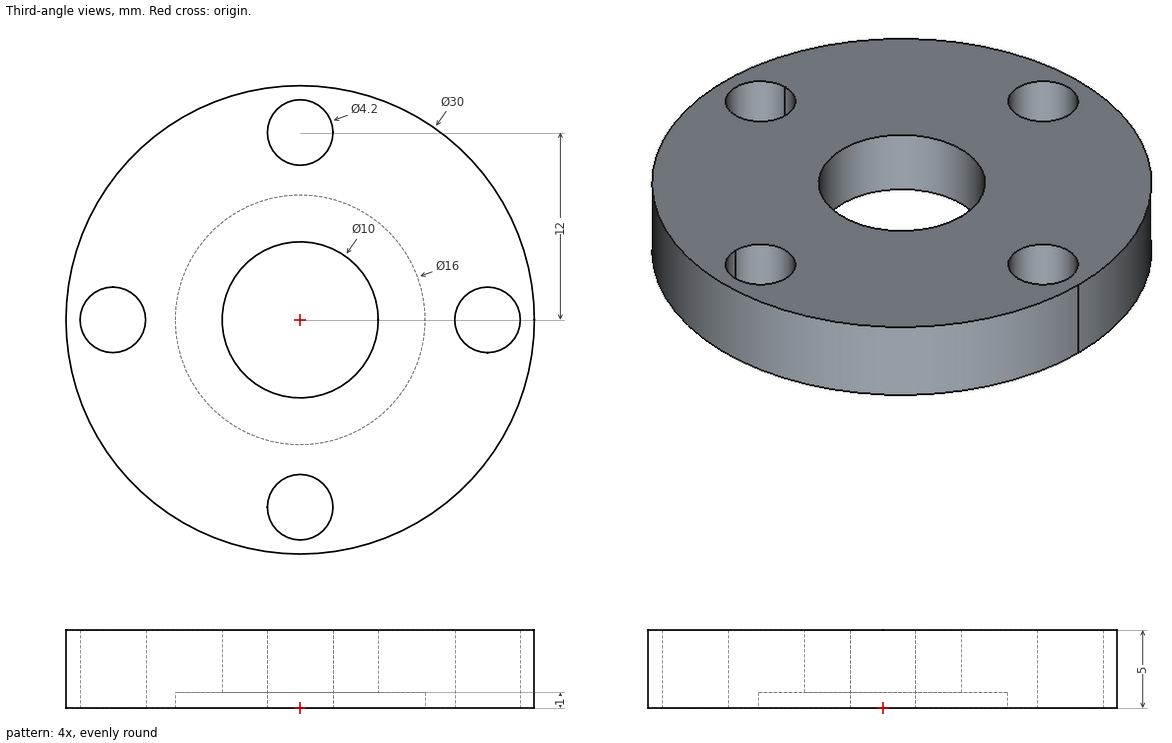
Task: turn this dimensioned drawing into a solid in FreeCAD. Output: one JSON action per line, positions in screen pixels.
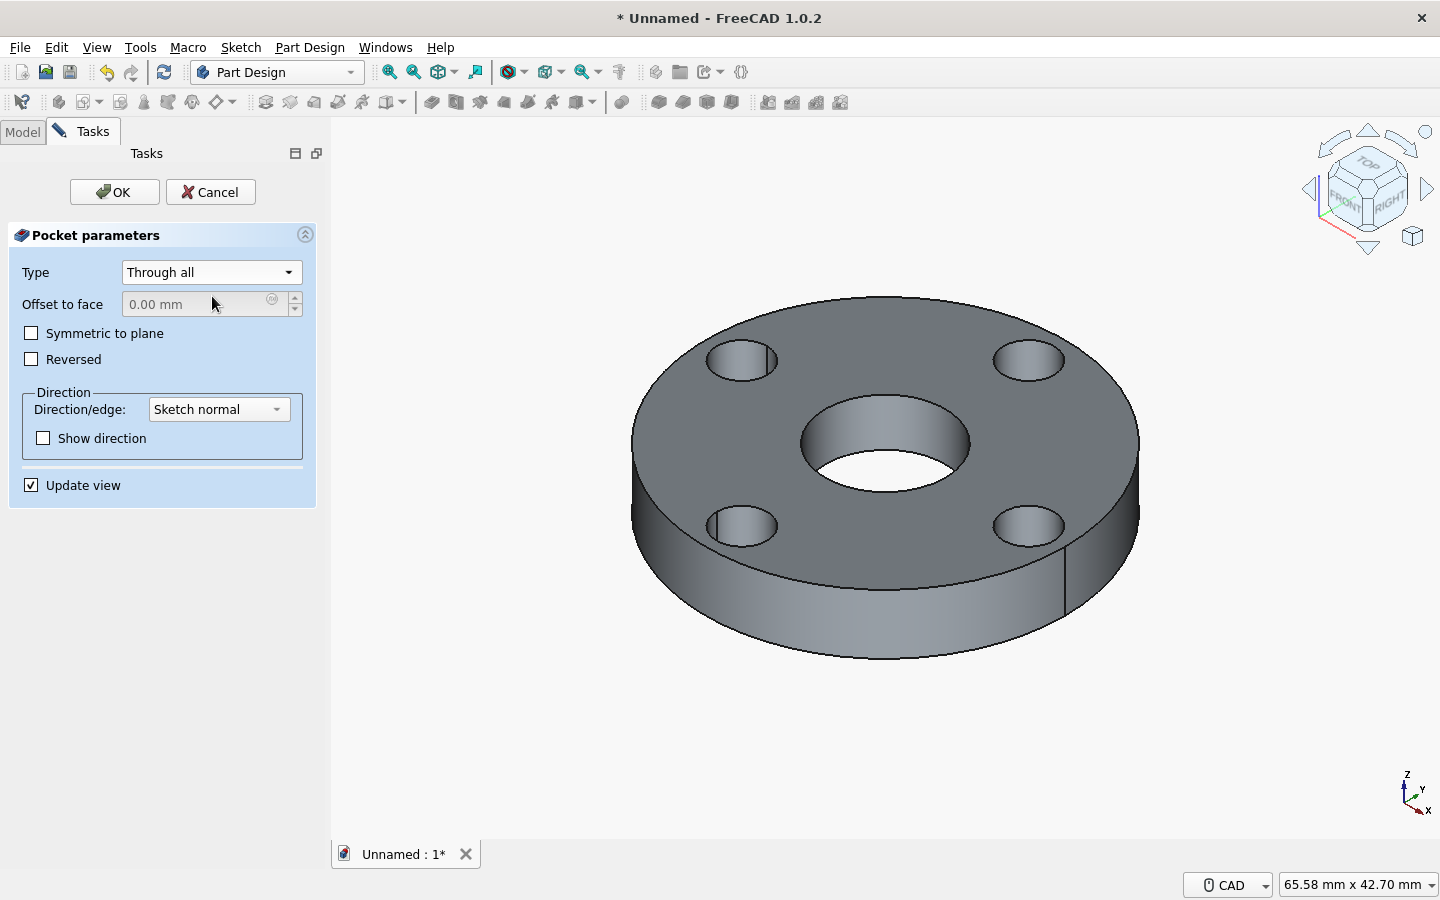
{"action": "left_click", "coordinate": [115, 192]}